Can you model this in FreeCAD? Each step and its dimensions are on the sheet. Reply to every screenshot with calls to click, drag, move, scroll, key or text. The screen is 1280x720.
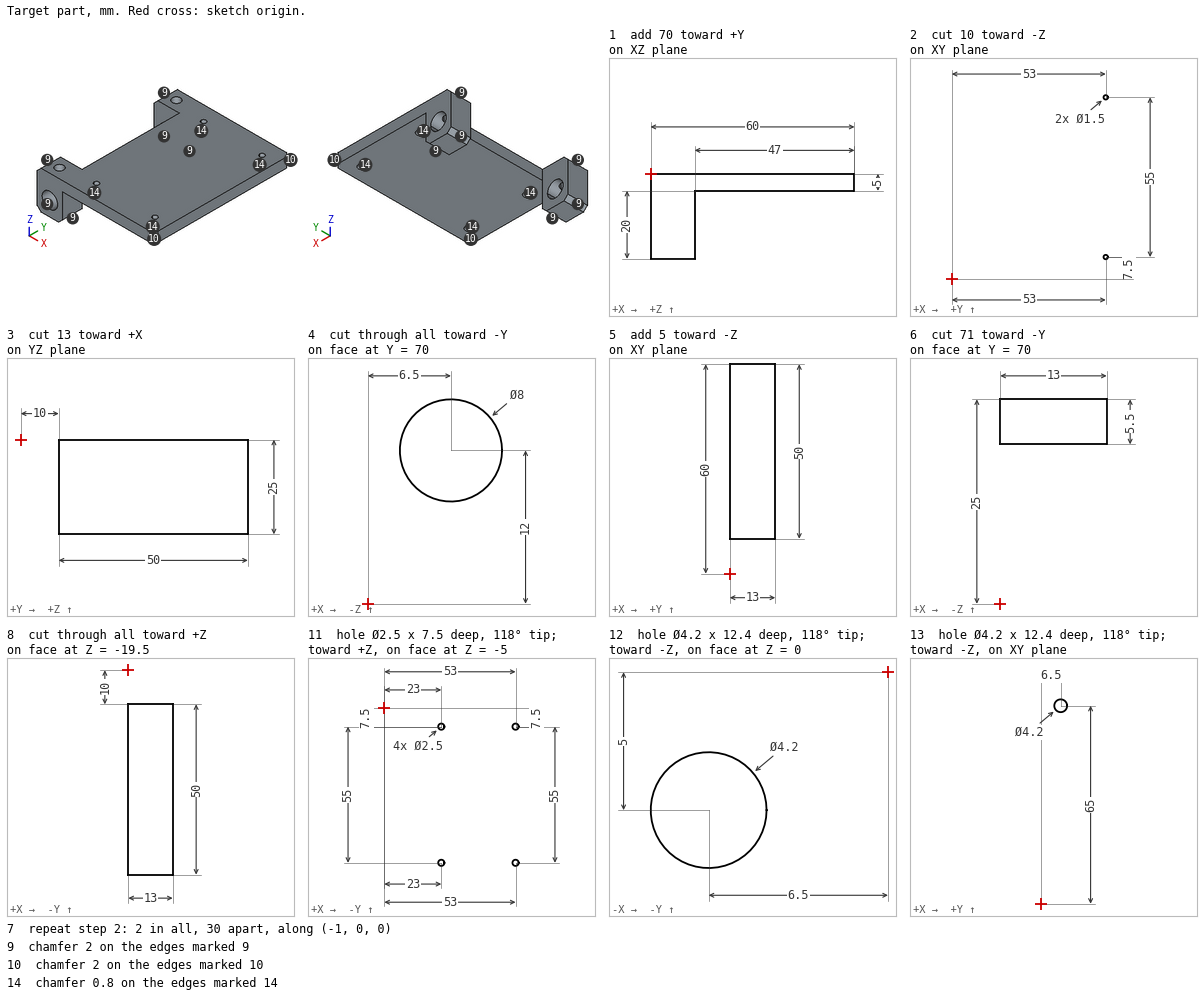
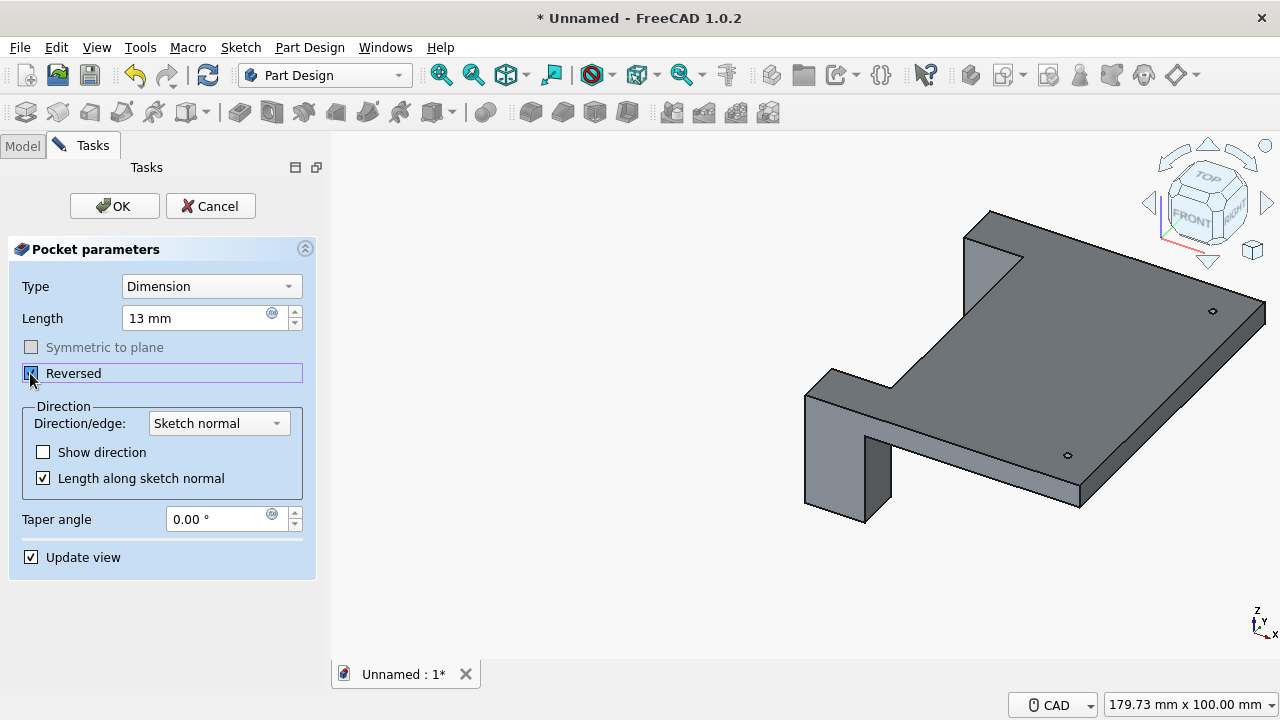
click(115, 206)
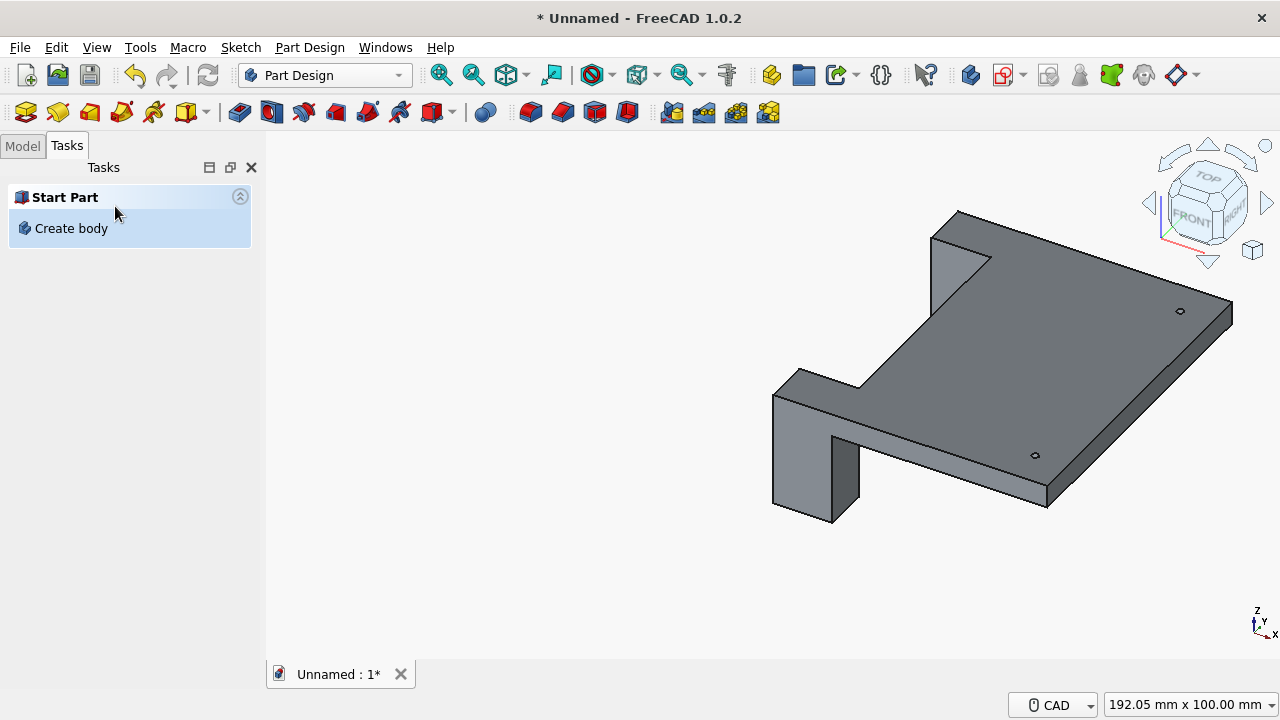
key(4)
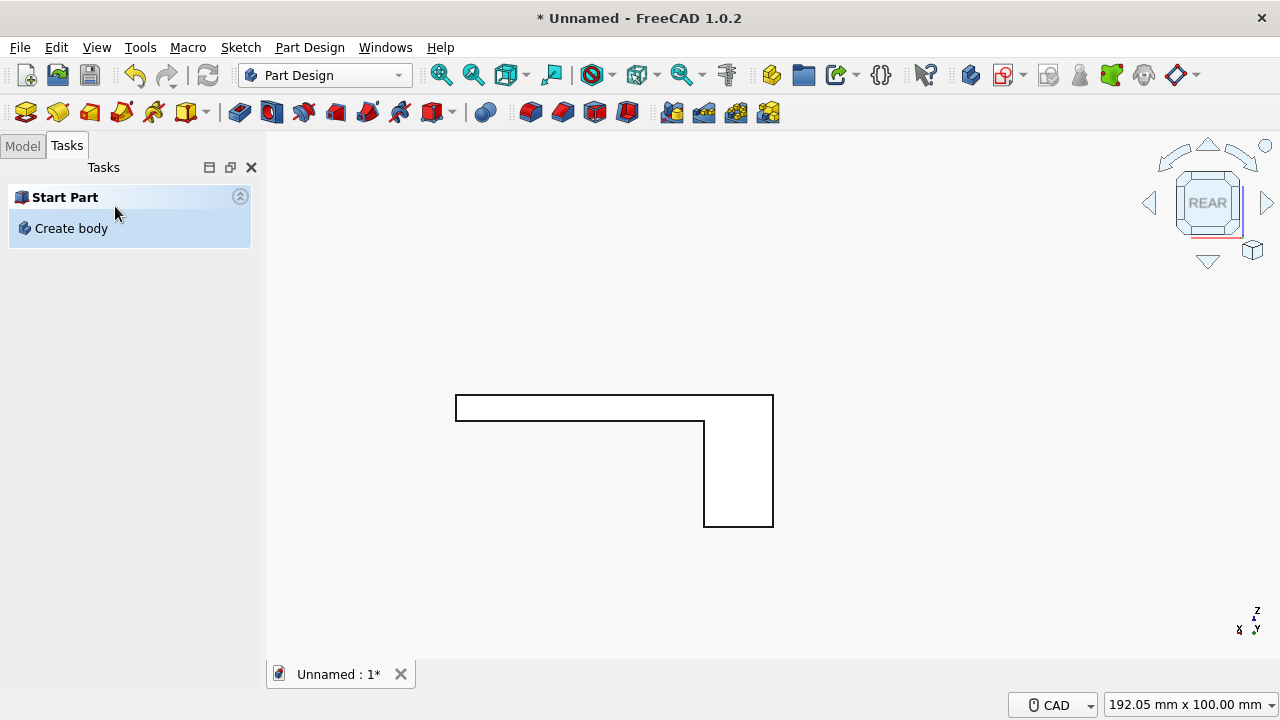
key(v)
key(f)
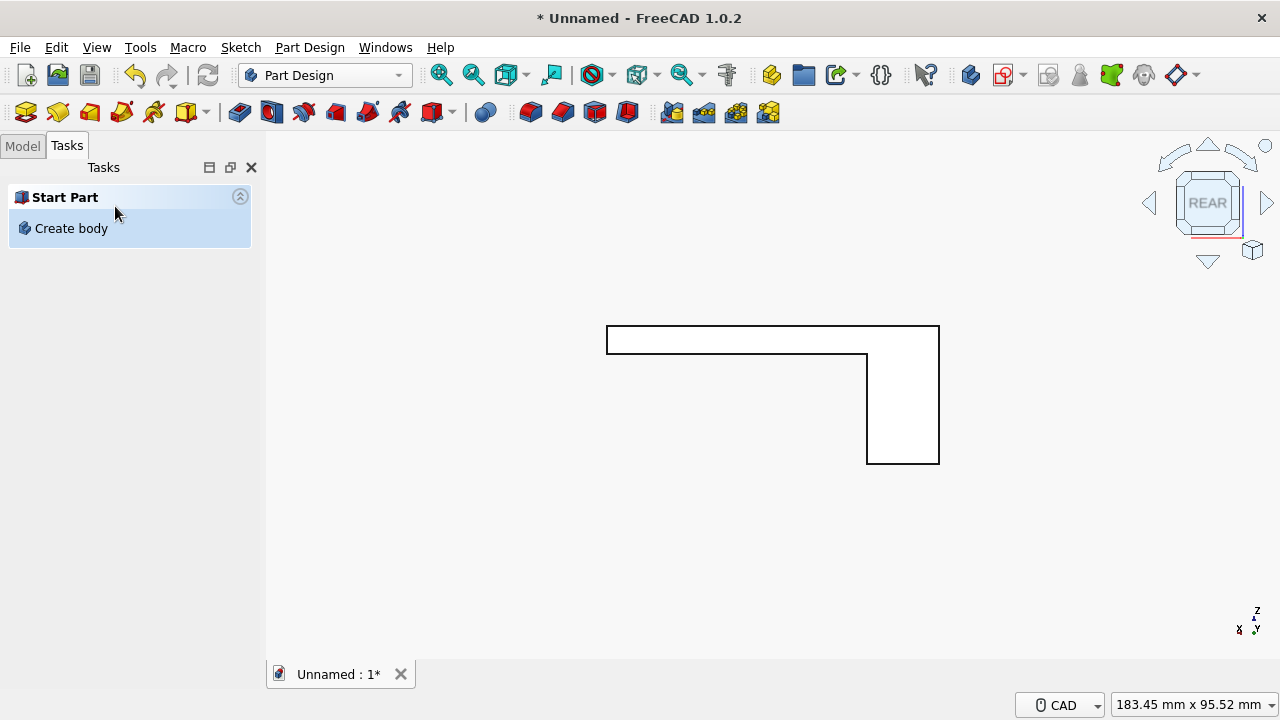
click(915, 355)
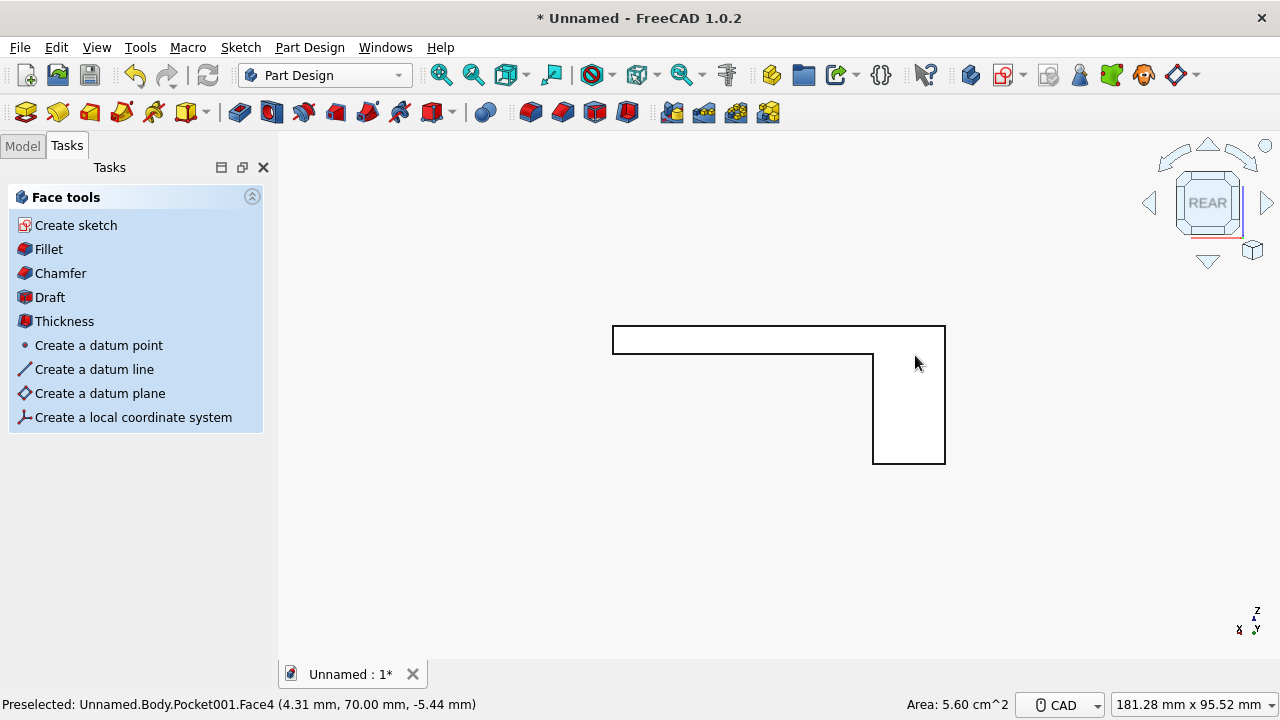
click(1004, 76)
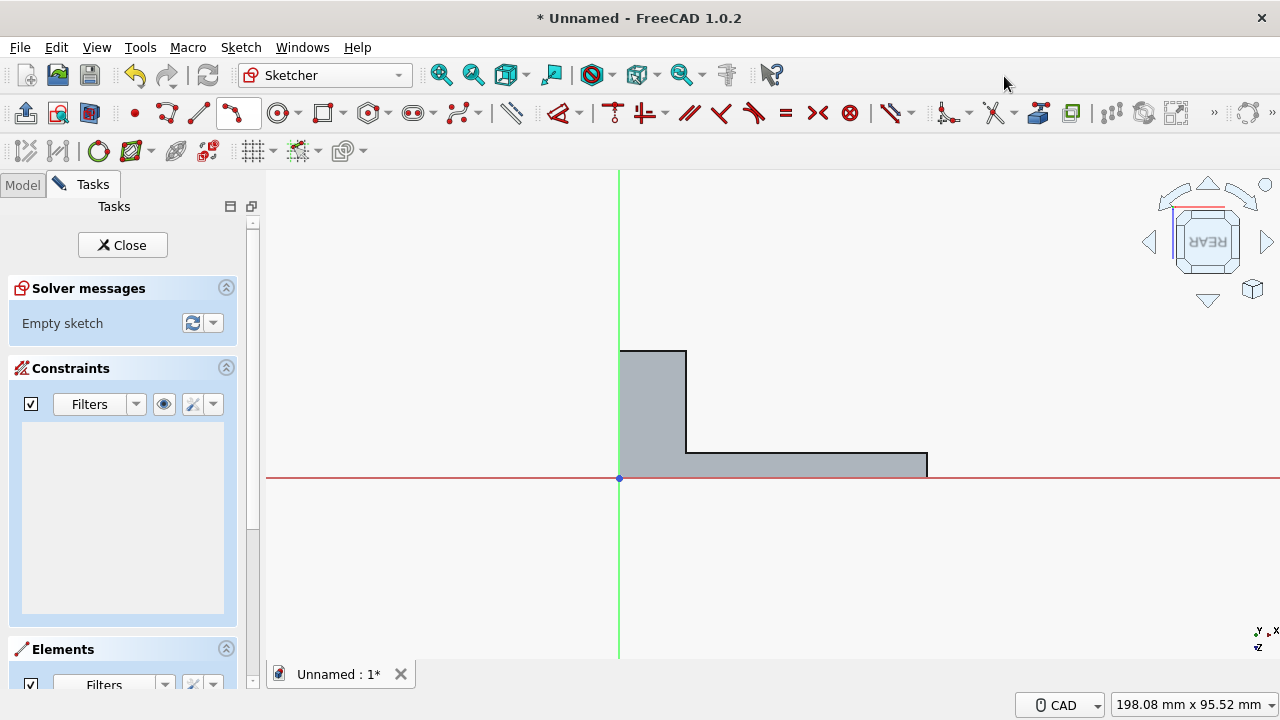
scroll(627, 445, up, 7)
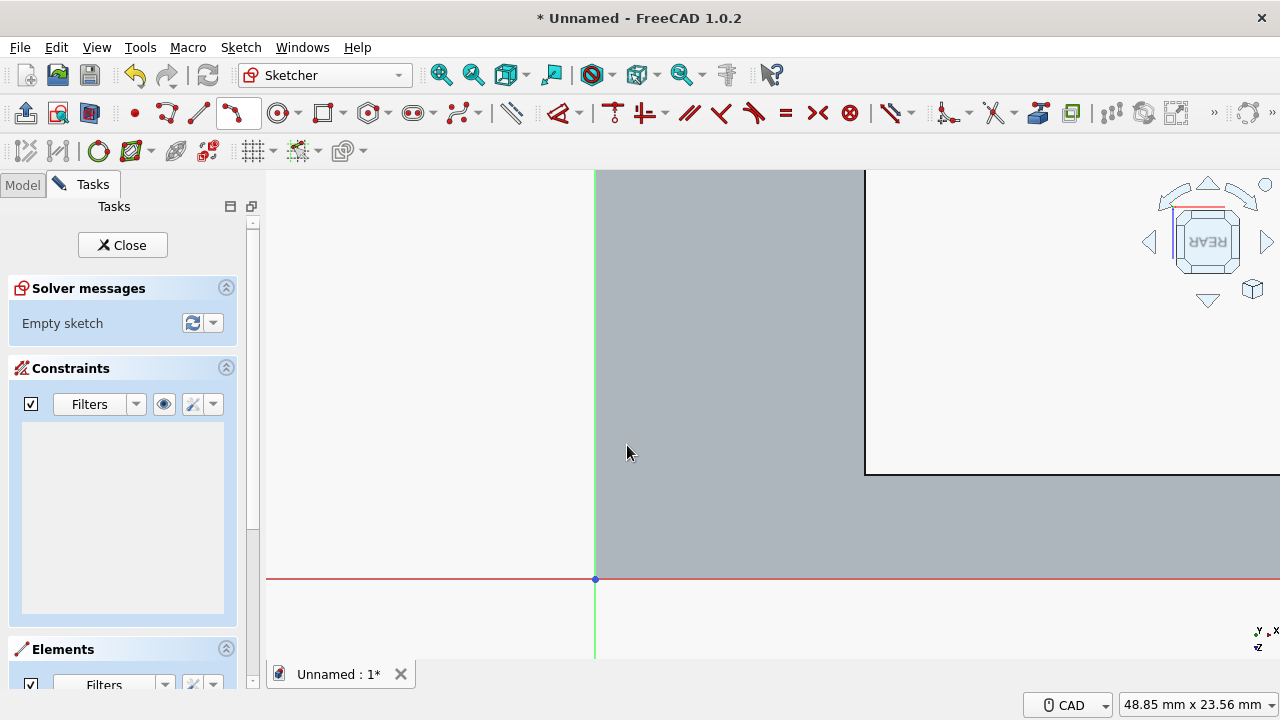
key(g)
key(c)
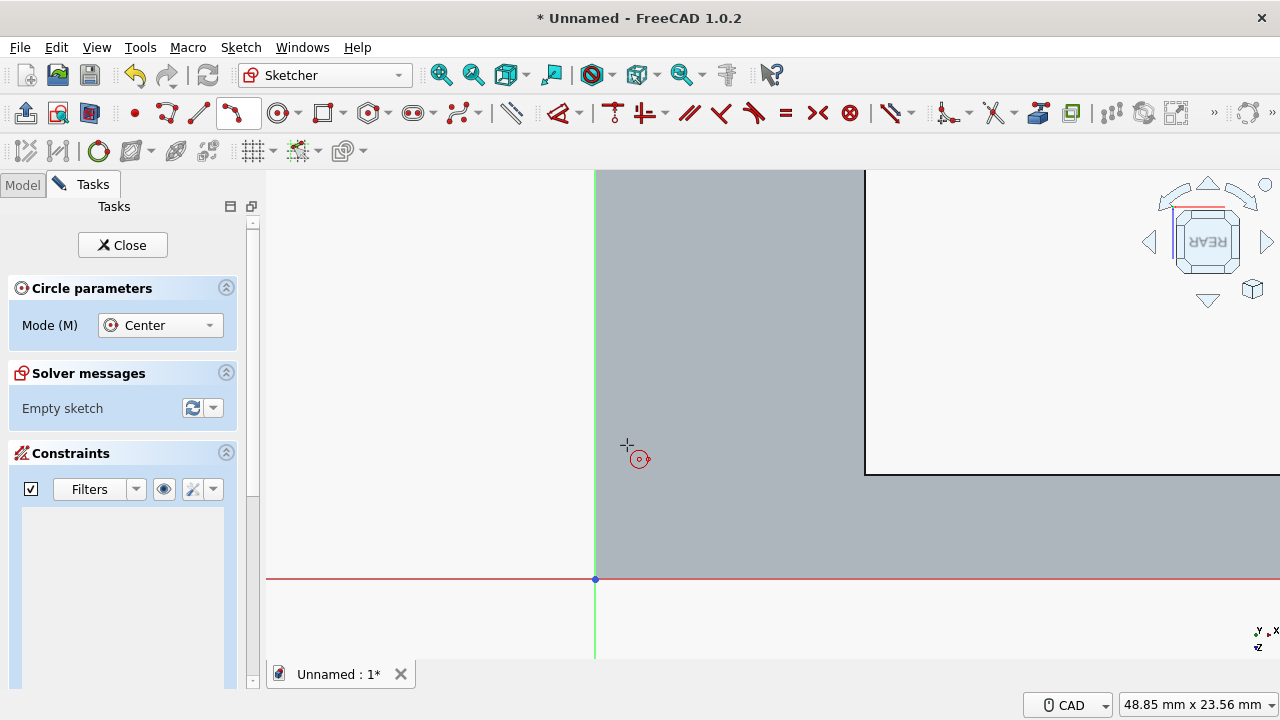
click(730, 330)
move(789, 271)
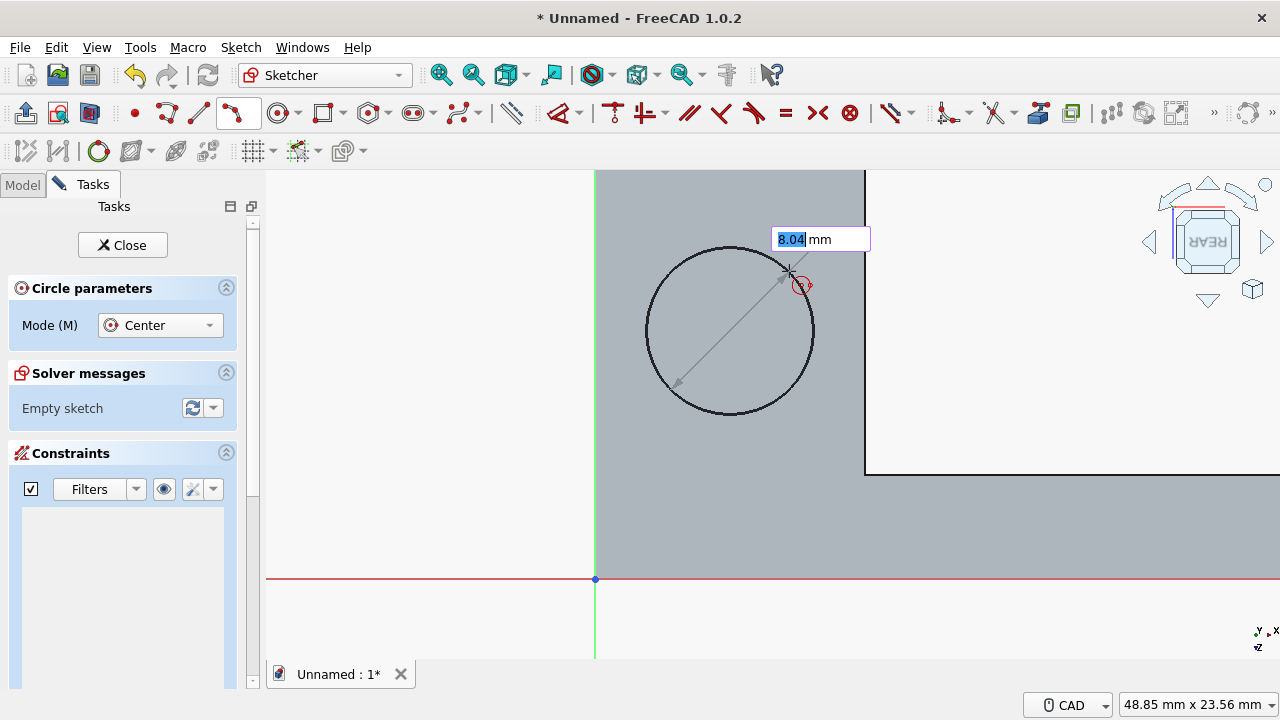
text(8)
key(Return)
key(Escape)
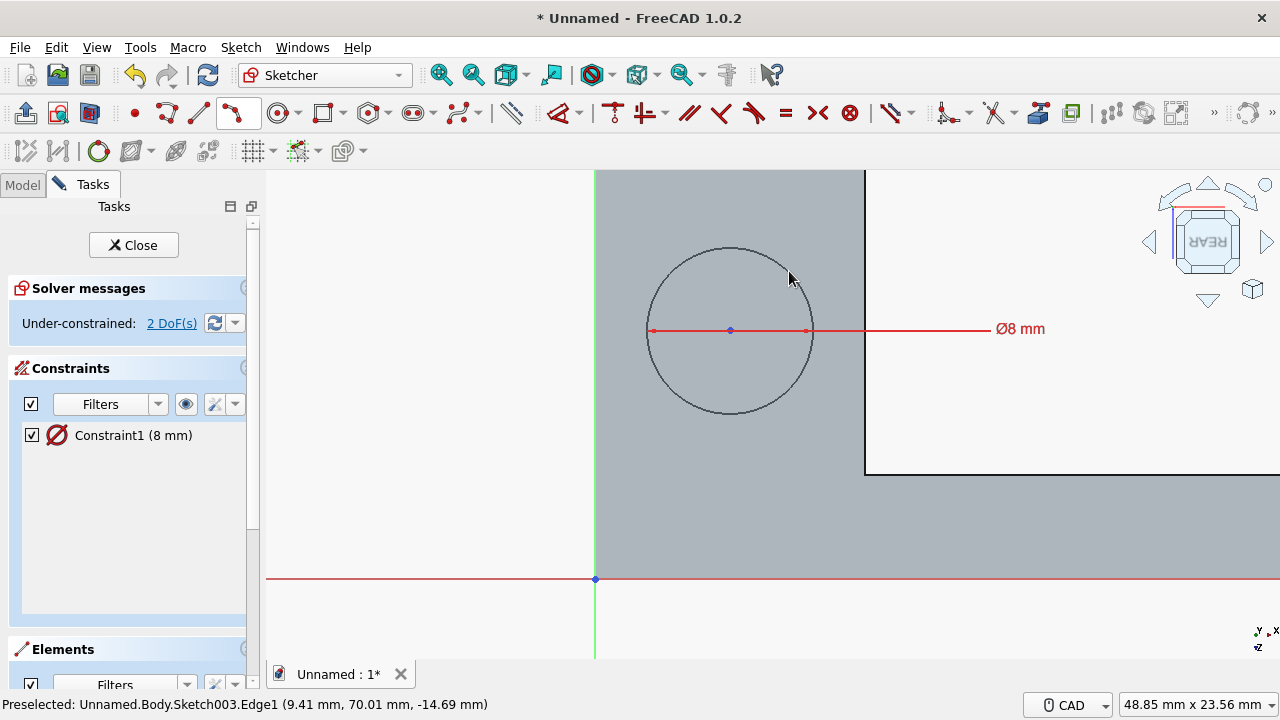
key(d)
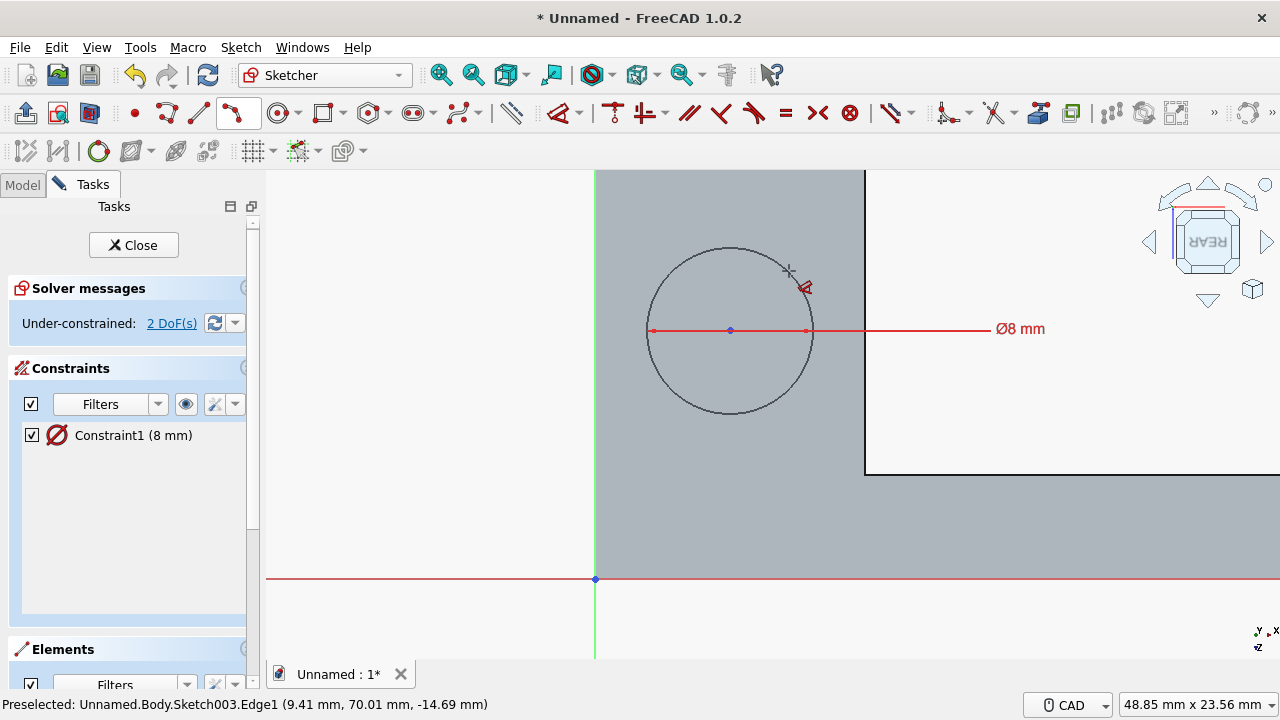
click(730, 331)
click(561, 455)